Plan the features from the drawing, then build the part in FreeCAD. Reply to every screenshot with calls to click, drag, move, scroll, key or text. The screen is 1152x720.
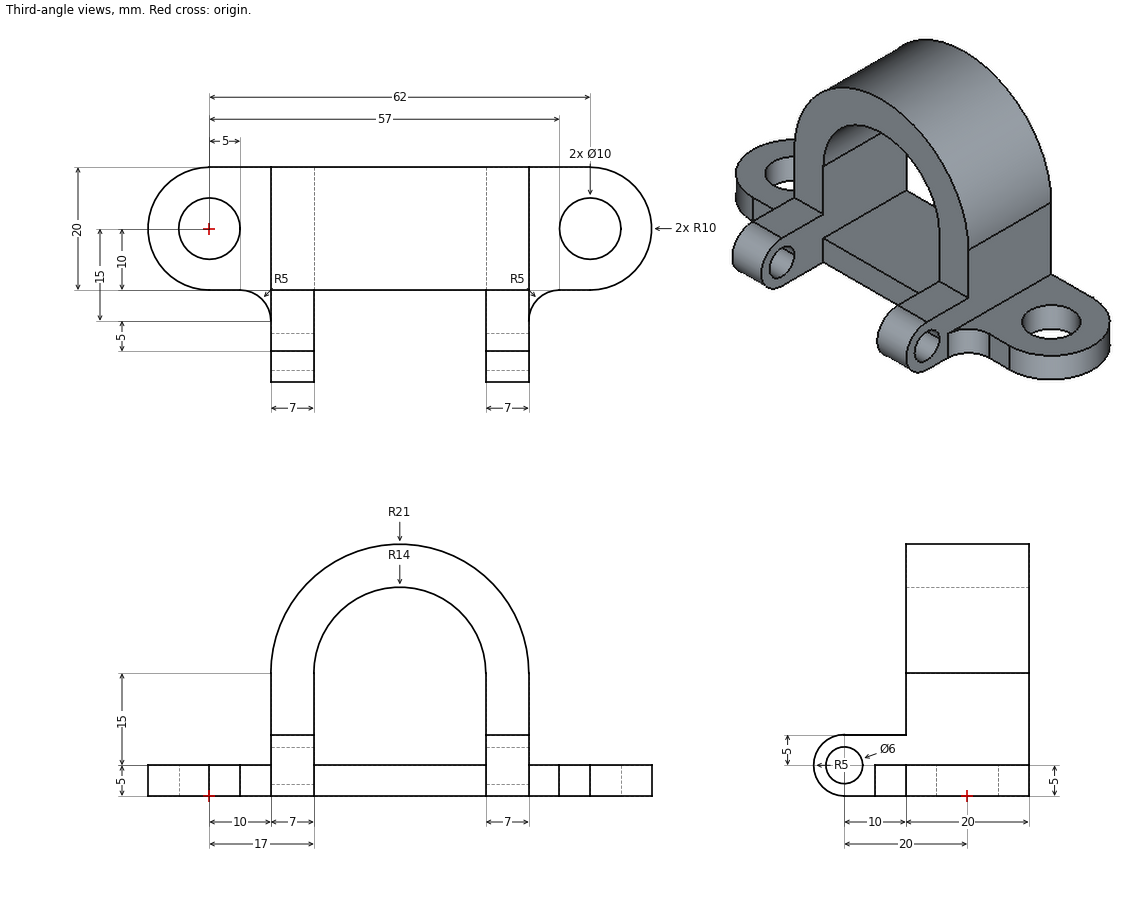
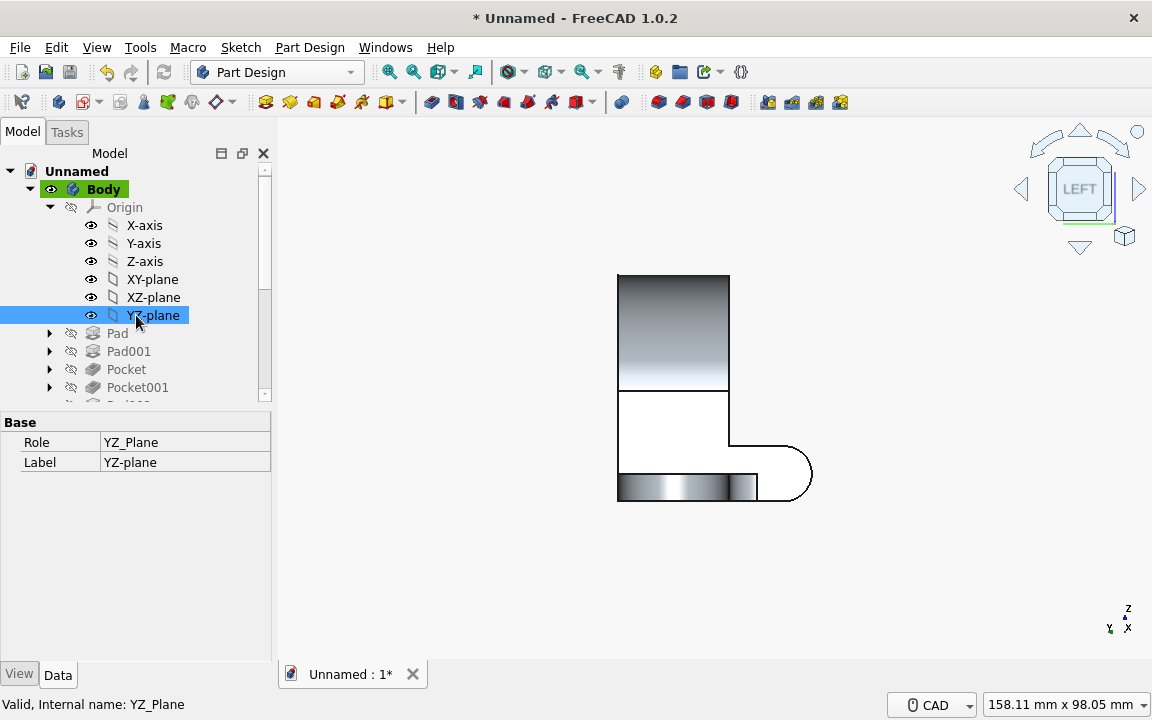
click(216, 102)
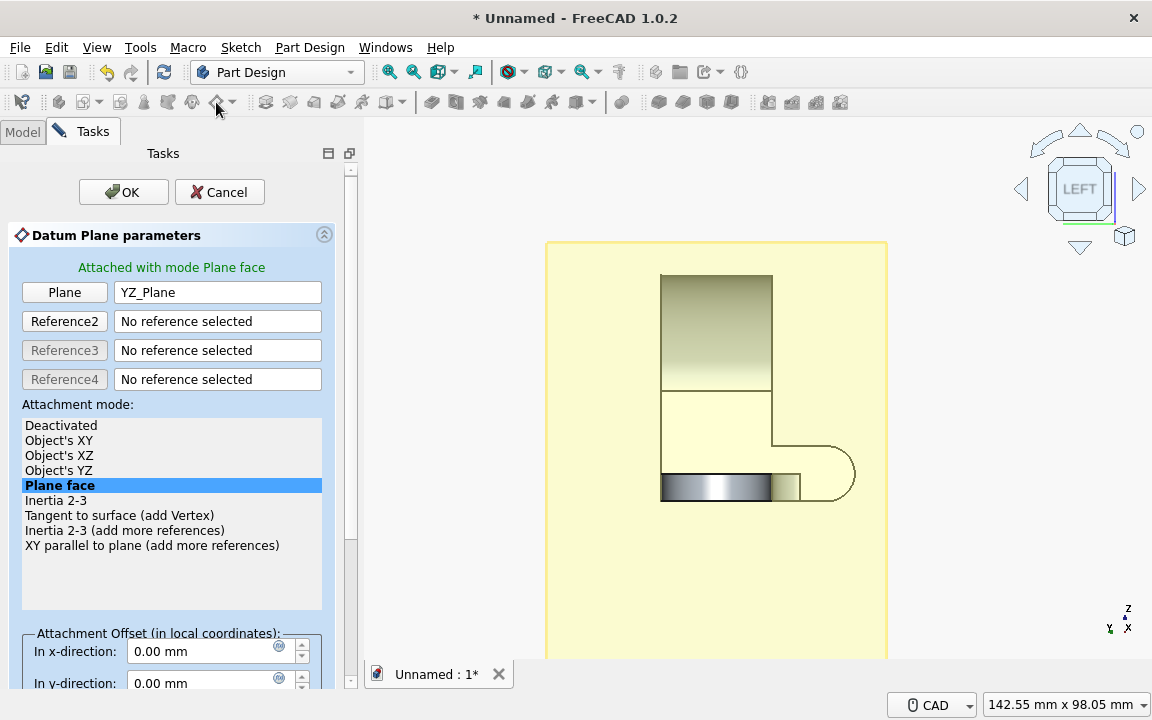
scroll(351, 426, down, 2)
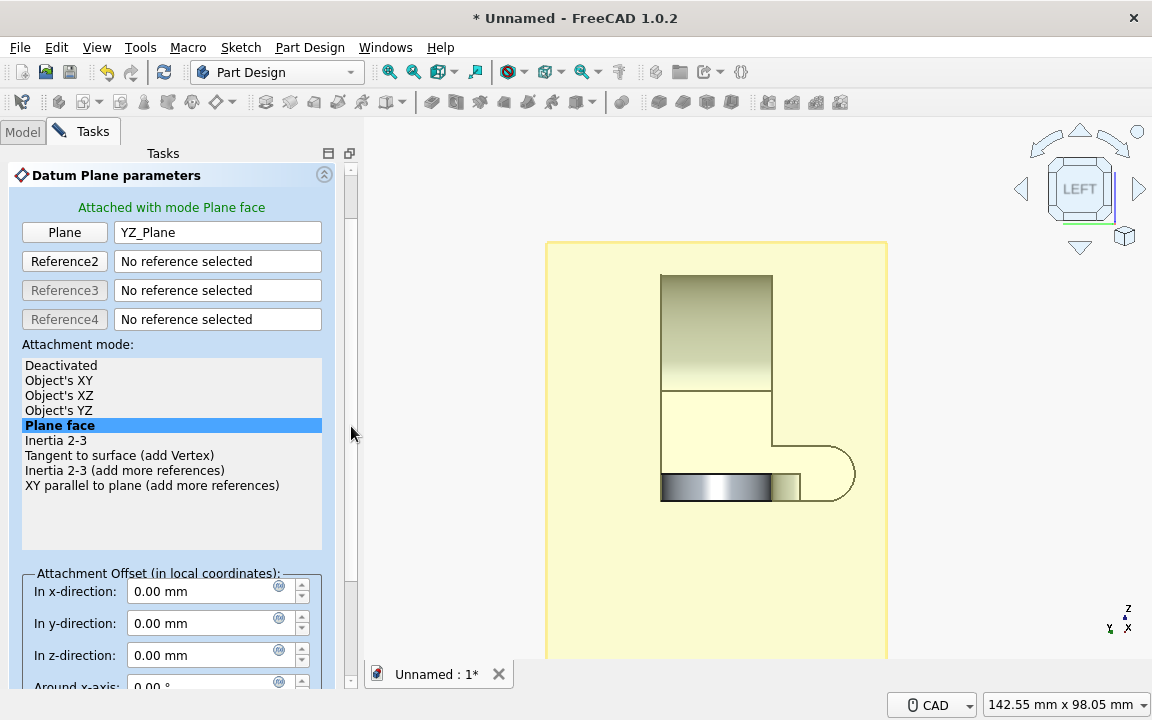
triple_click(210, 595)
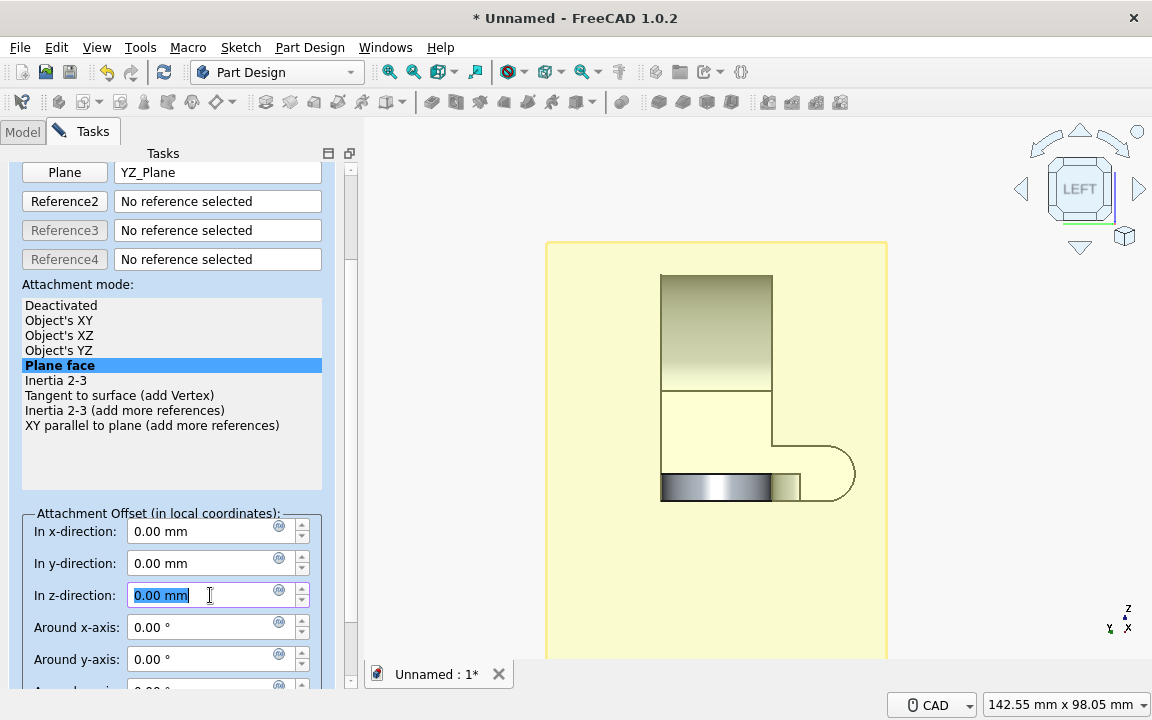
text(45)
key(Tab)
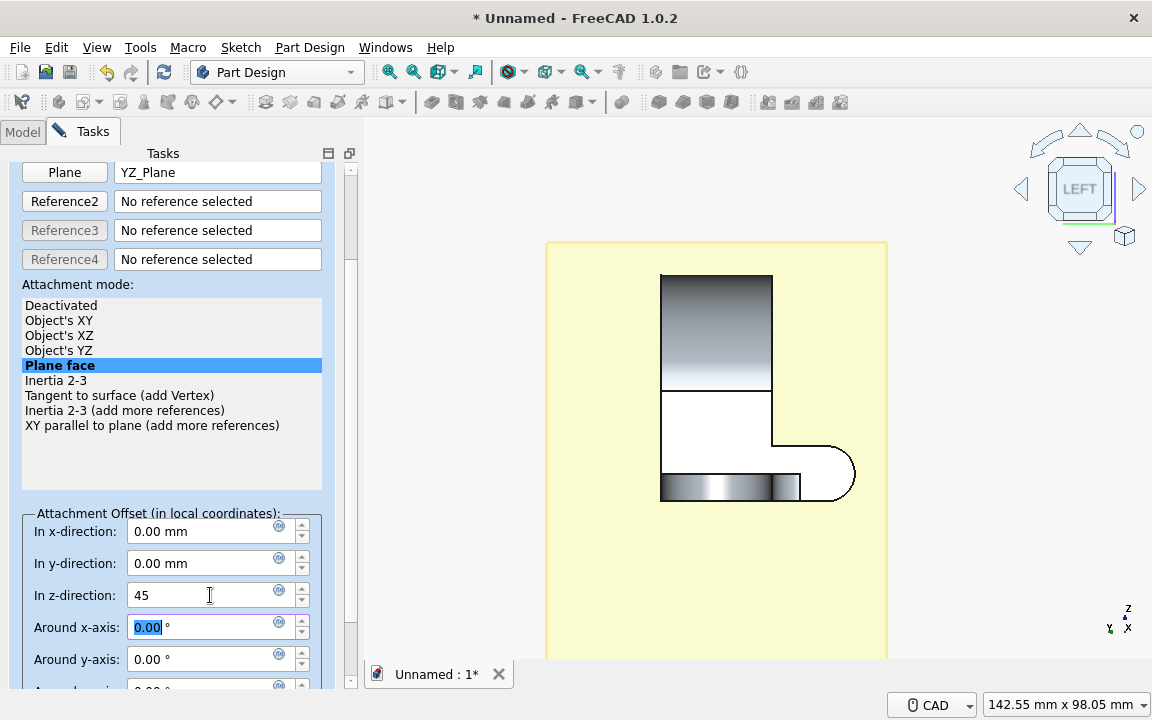
scroll(351, 426, up, 3)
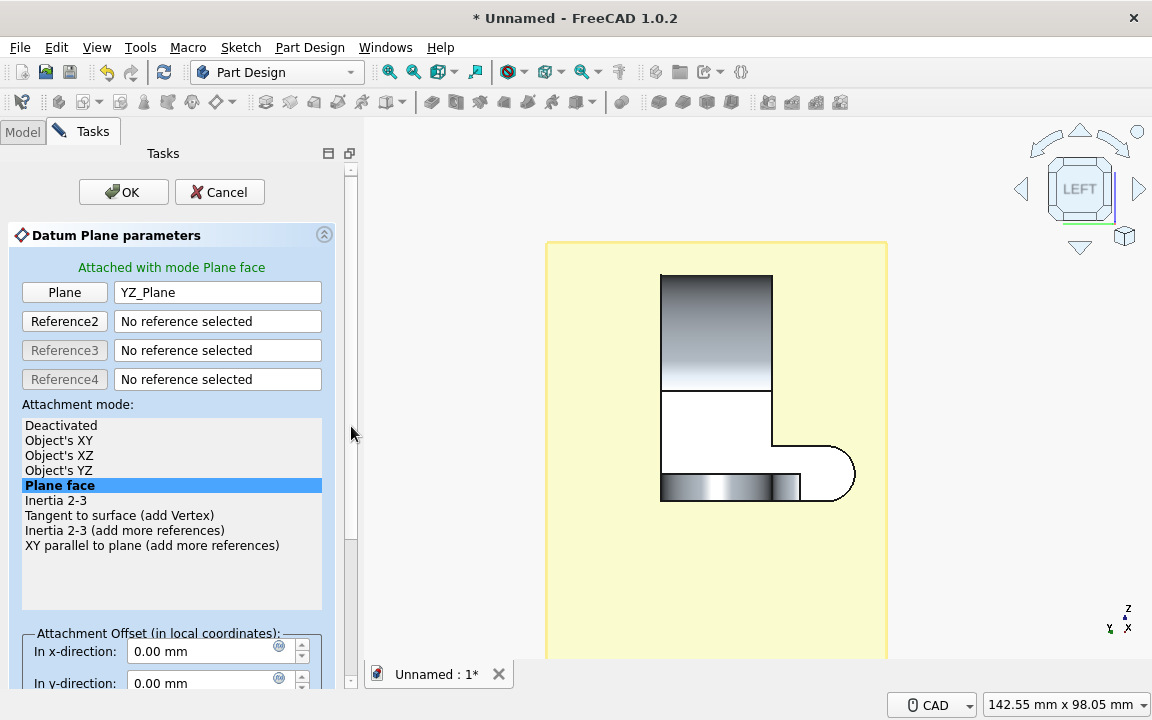
click(124, 192)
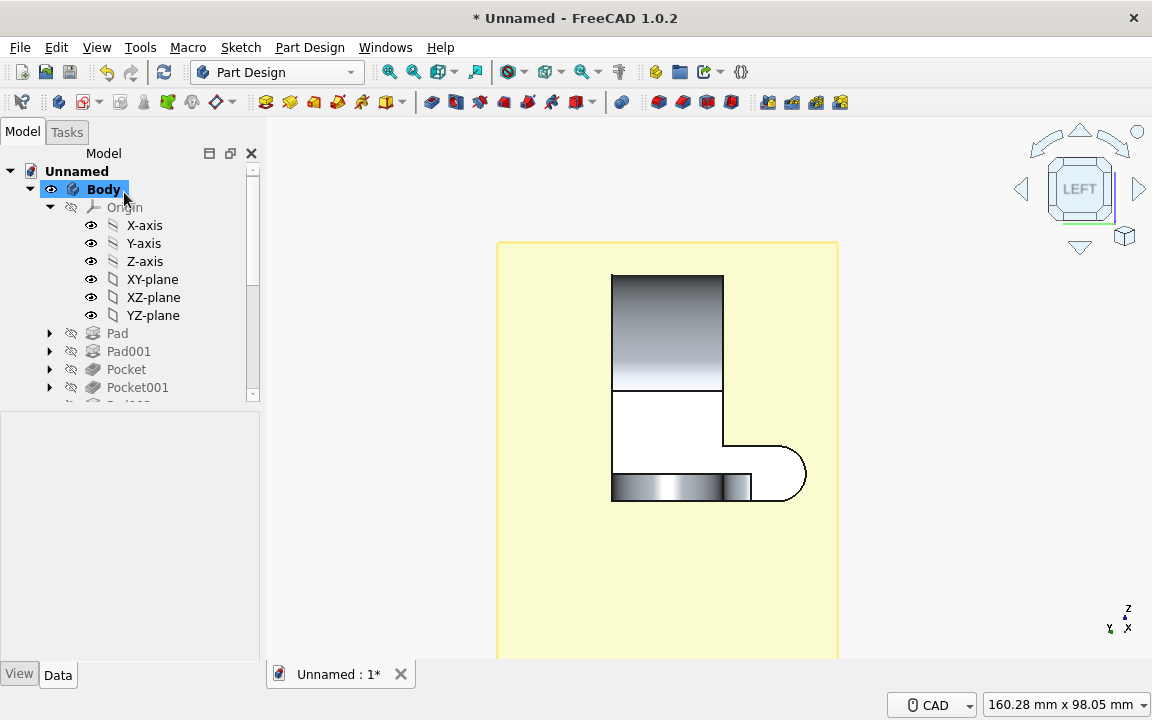
scroll(100, 275, down, 3)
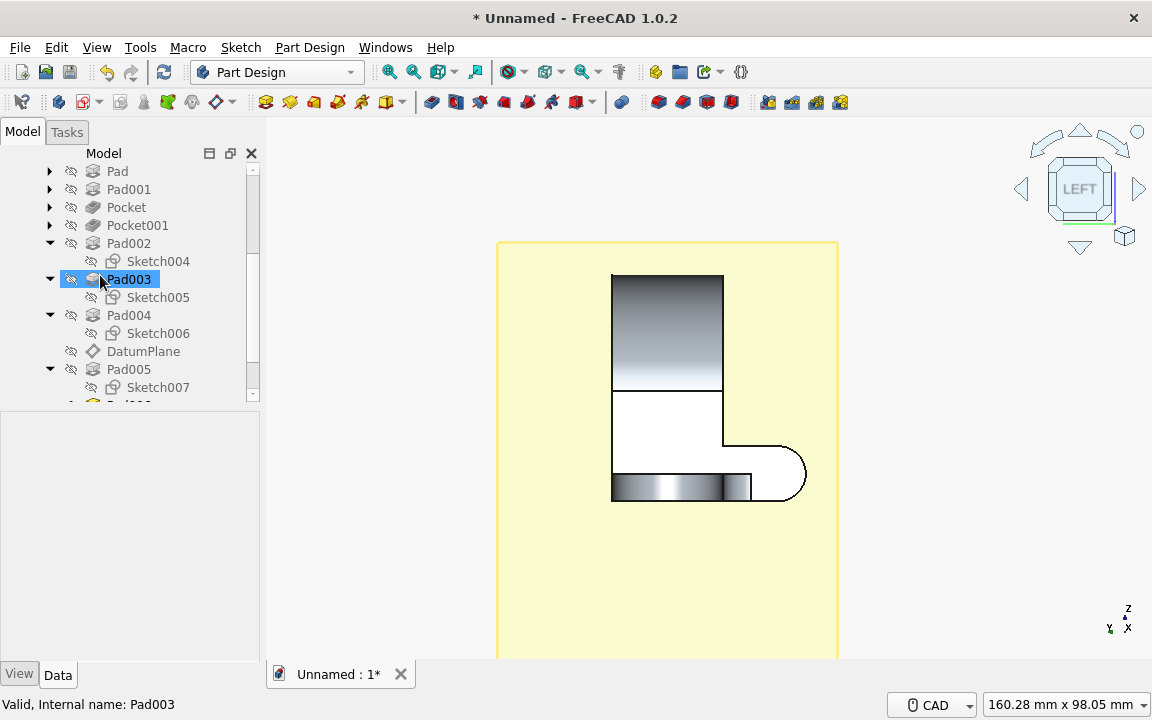
scroll(140, 275, up, 15)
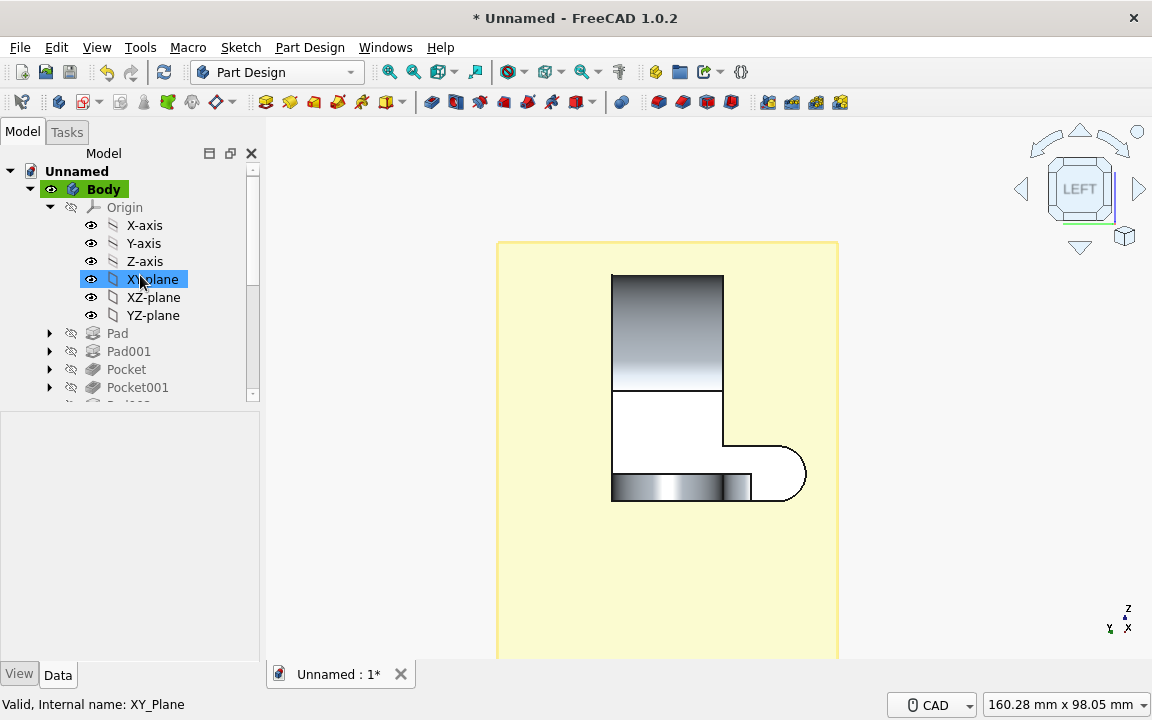
scroll(100, 275, down, 6)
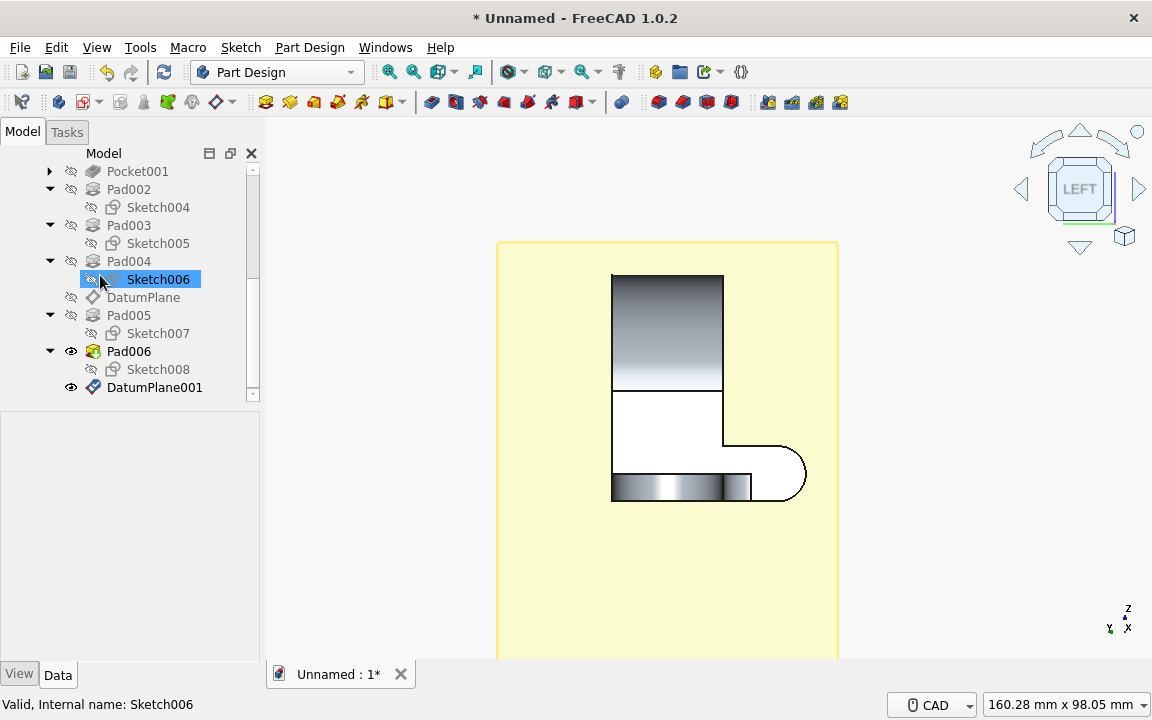
click(116, 387)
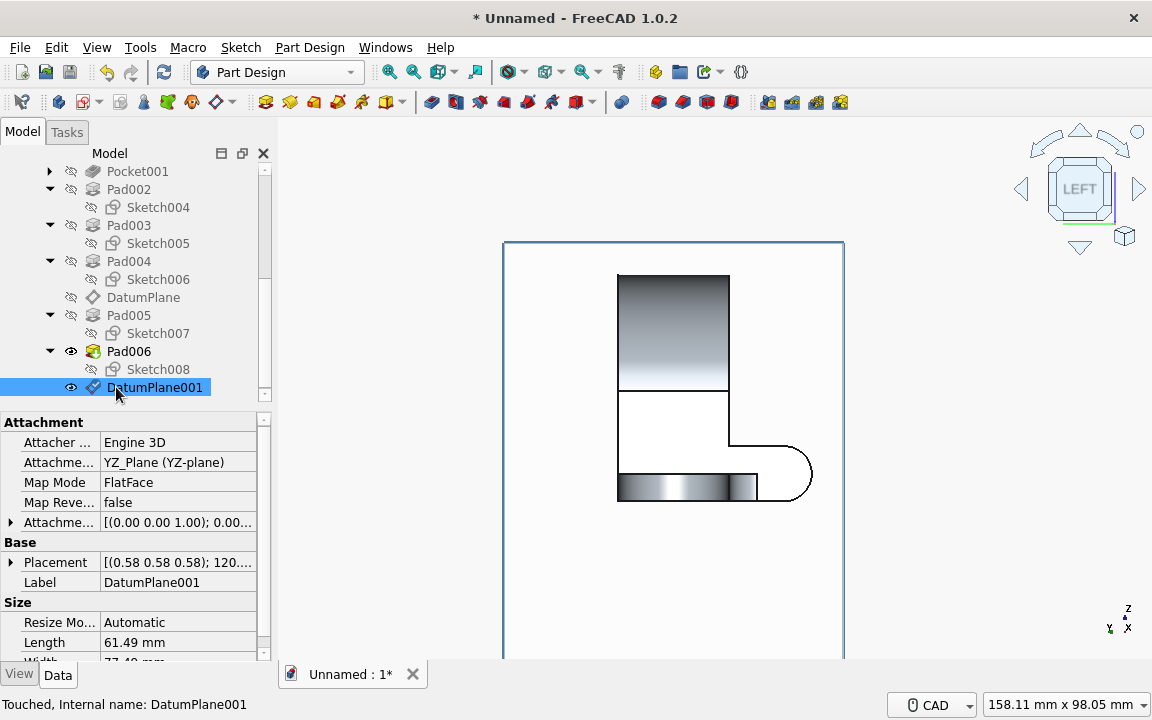
click(84, 102)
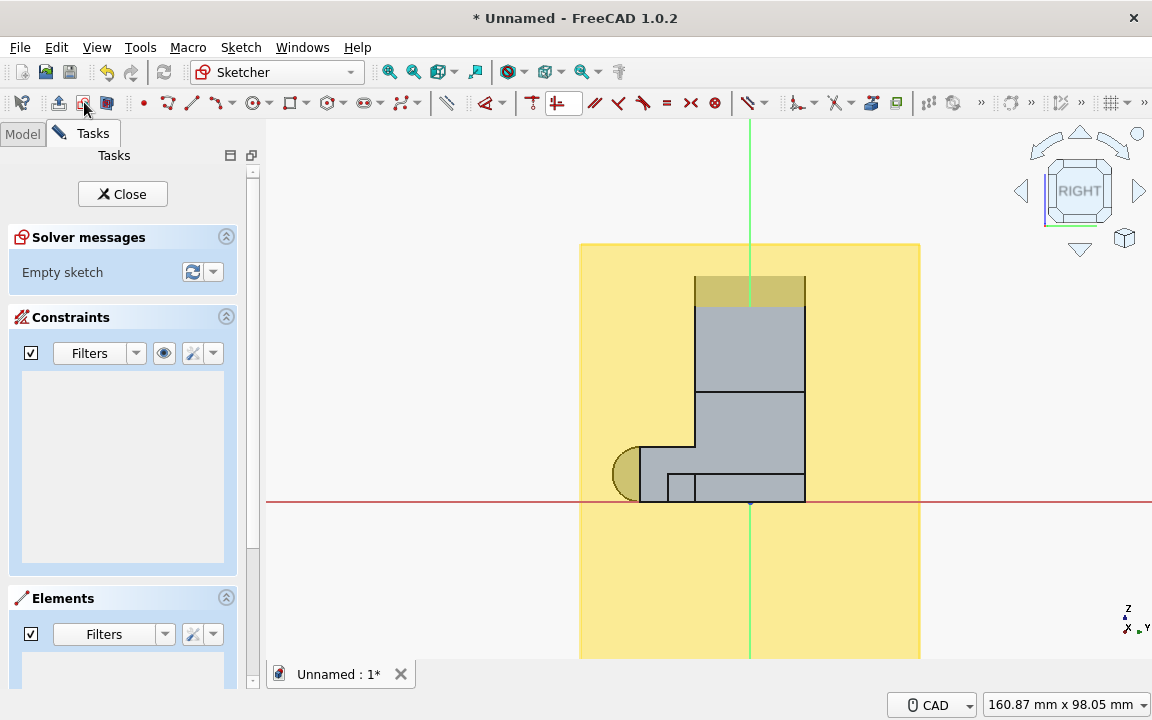
key(q)
key(s)